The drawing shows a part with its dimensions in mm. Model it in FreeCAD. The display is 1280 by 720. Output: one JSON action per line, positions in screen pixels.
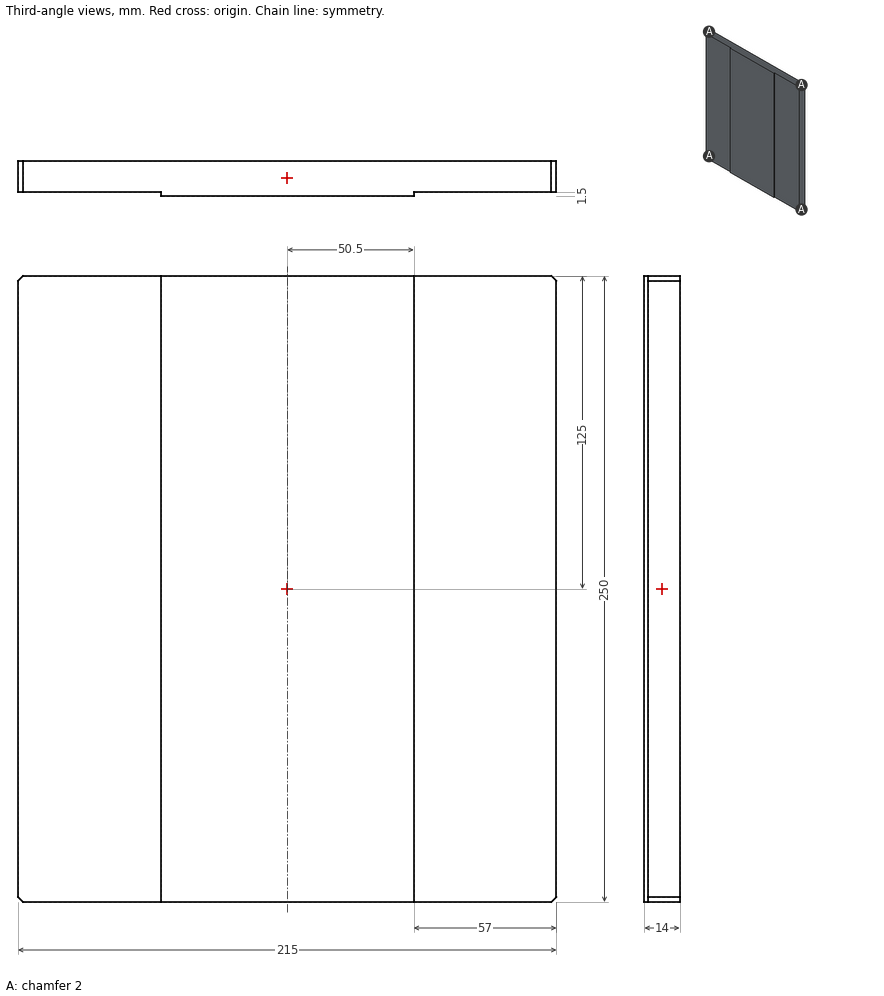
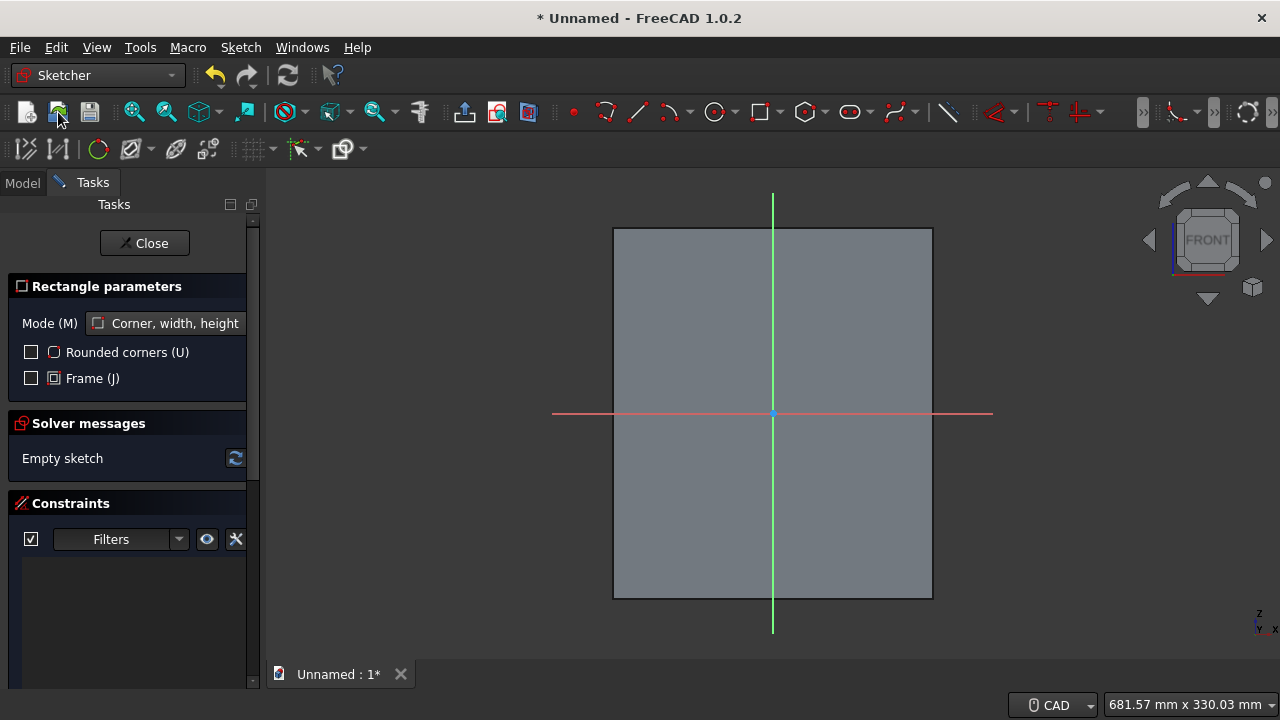
{"action": "left_click", "coordinate": [848, 228]}
{"action": "left_click", "coordinate": [933, 599]}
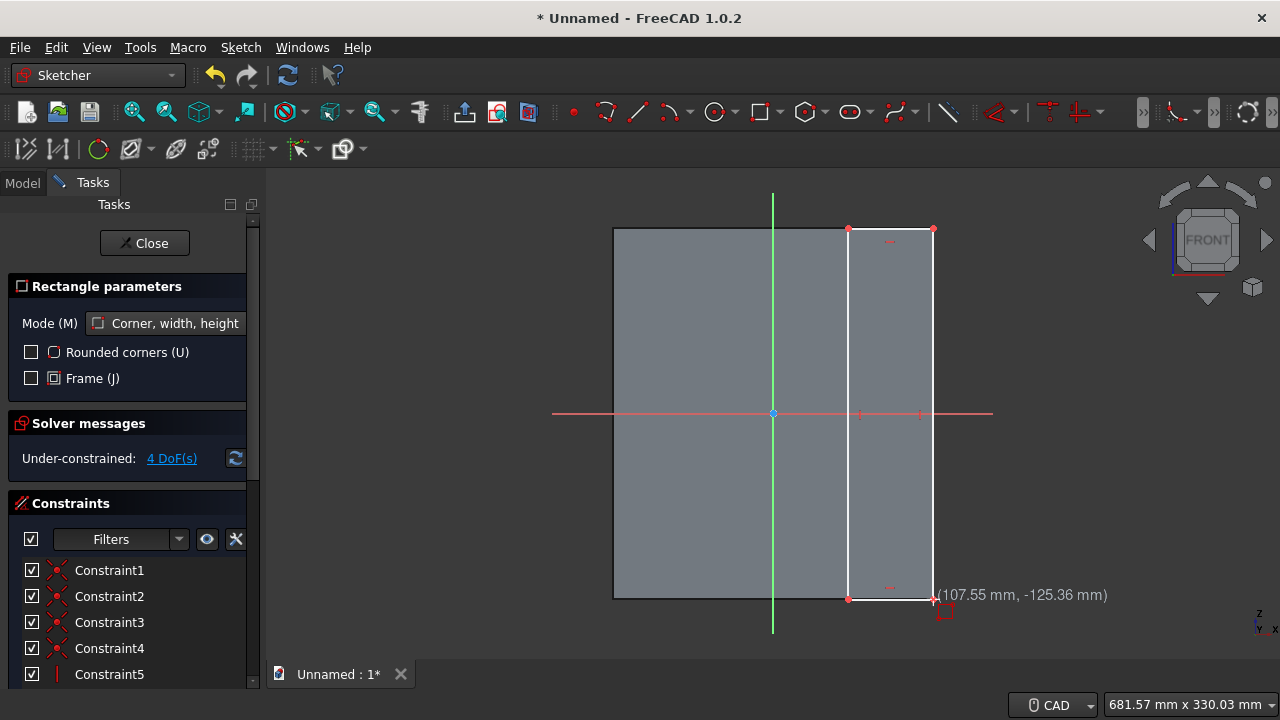
{"action": "left_click", "coordinate": [613, 228]}
{"action": "left_click", "coordinate": [698, 599]}
{"action": "key", "text": "Escape"}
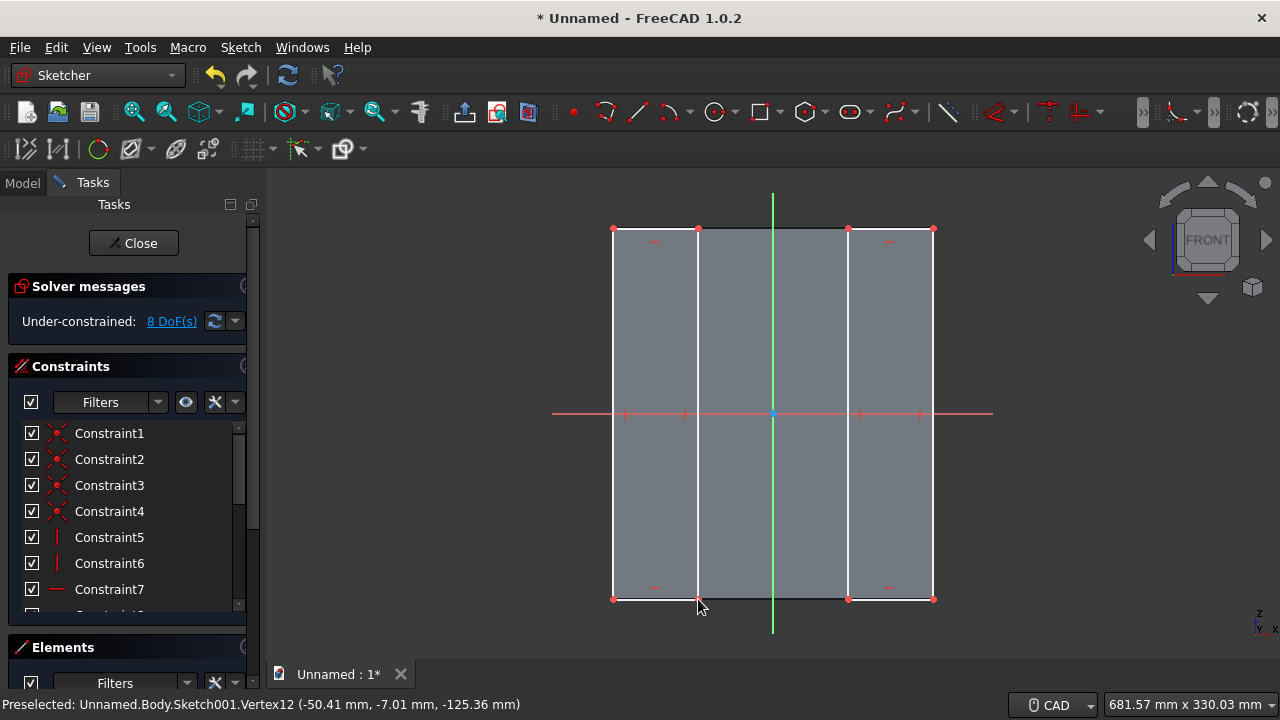
{"action": "left_click", "coordinate": [933, 229]}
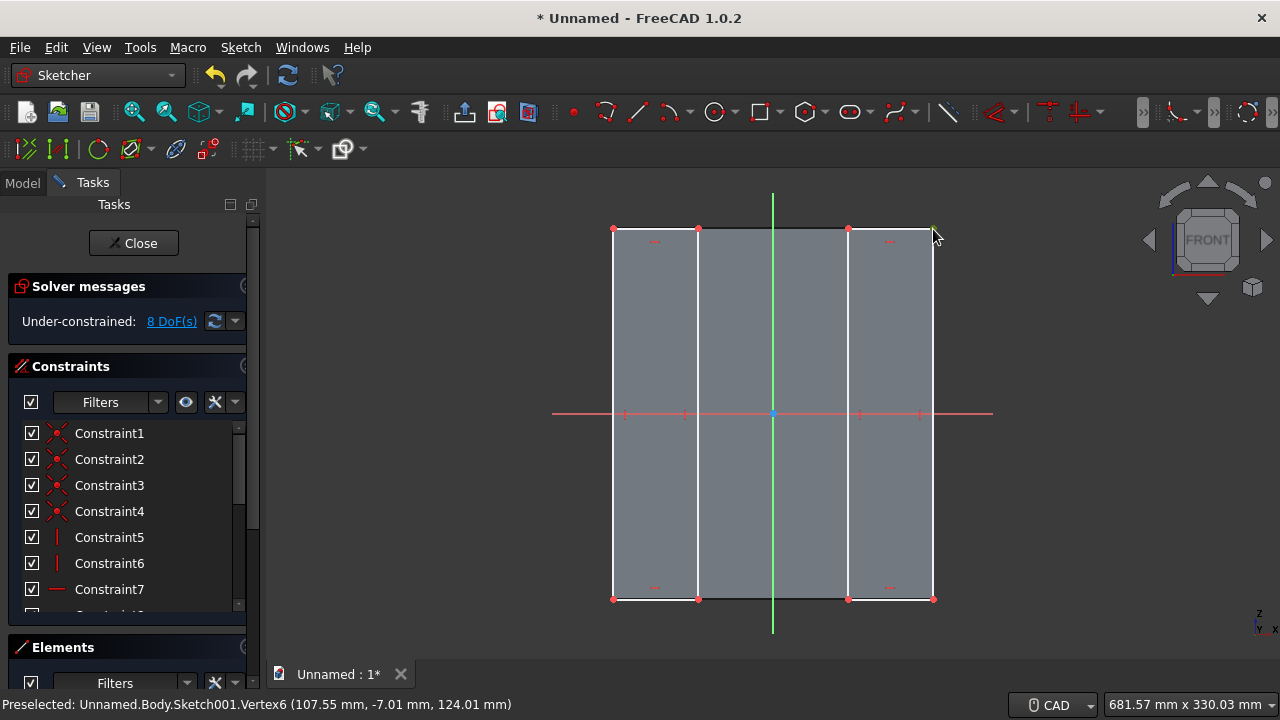
{"action": "left_click", "coordinate": [613, 229]}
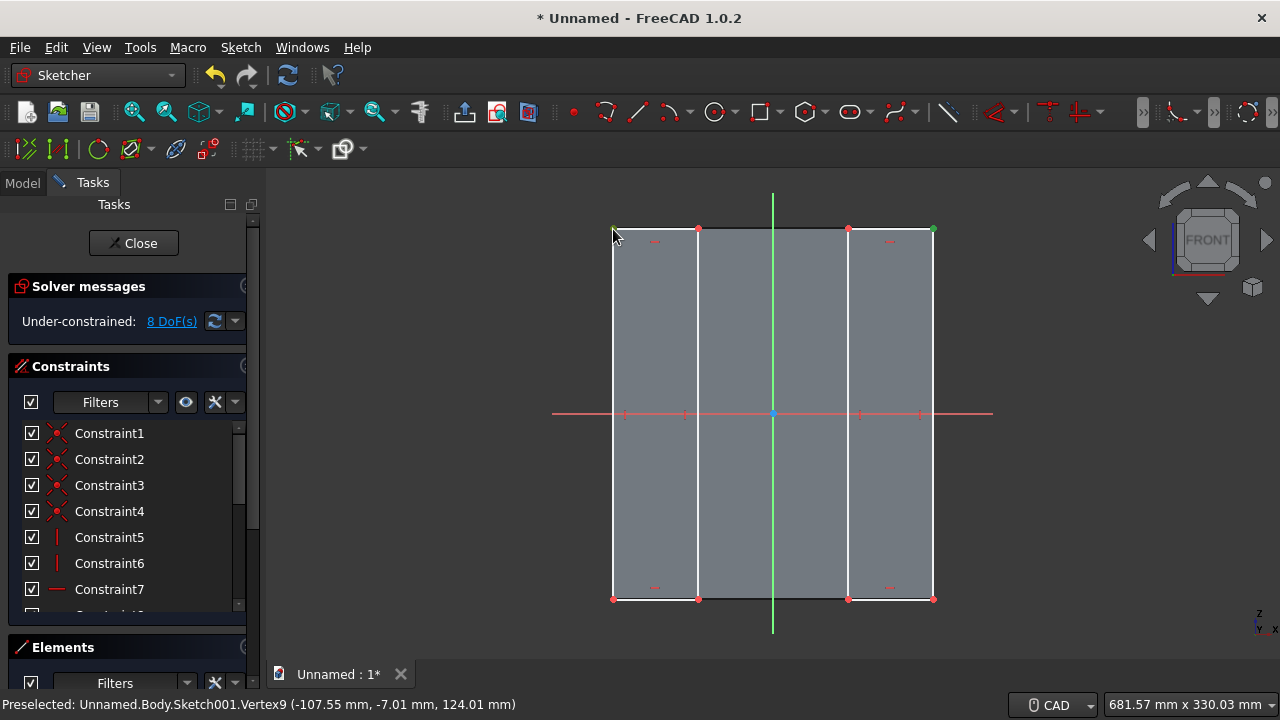
{"action": "left_click", "coordinate": [773, 600]}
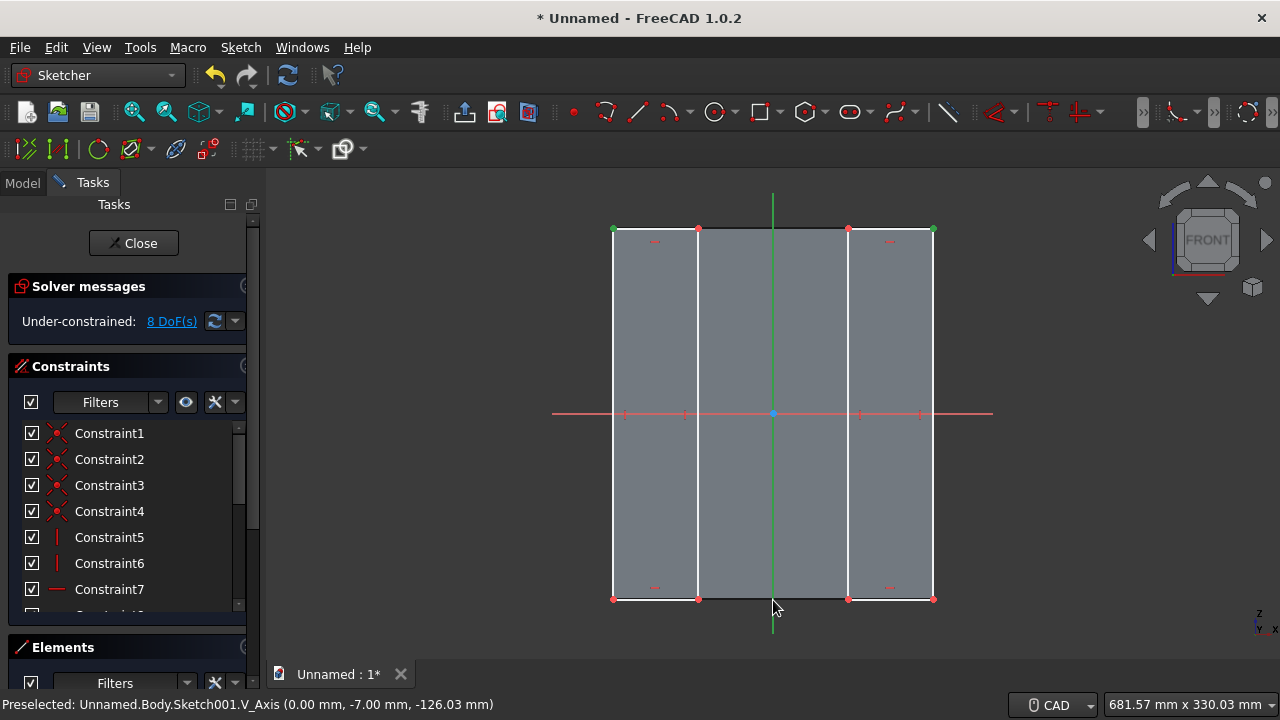
{"action": "key", "text": "s"}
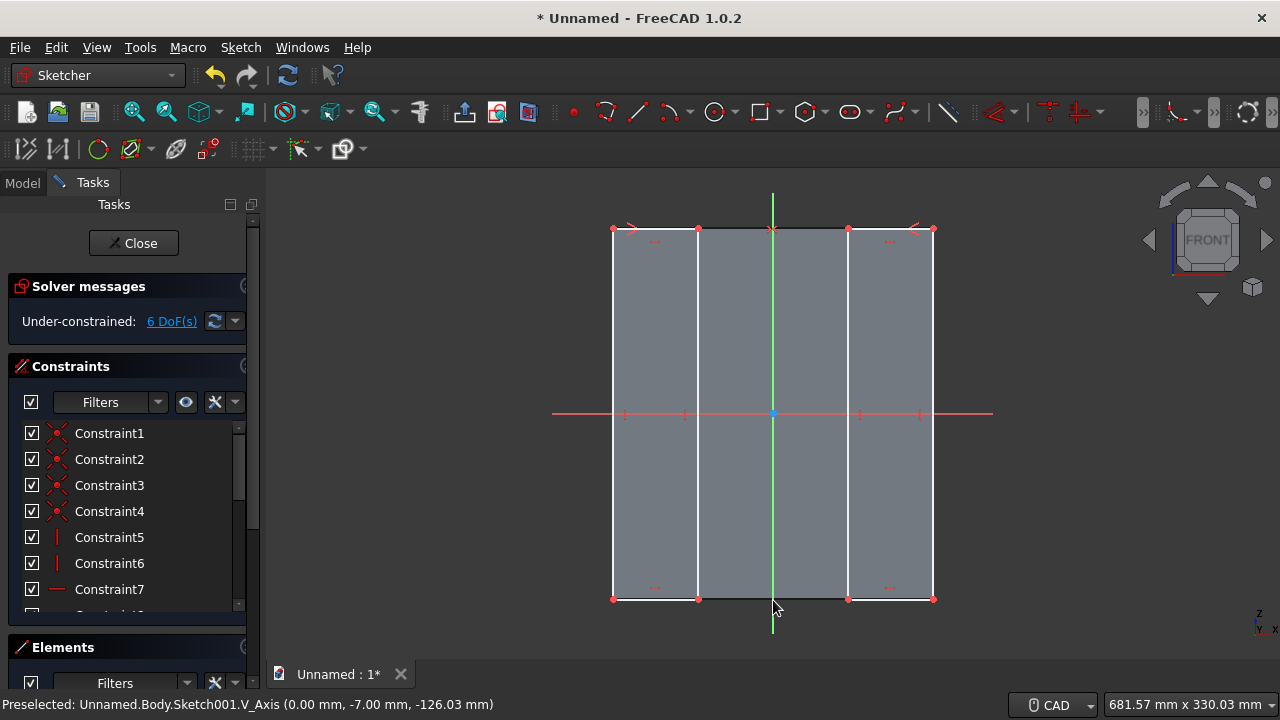
{"action": "left_click", "coordinate": [848, 600]}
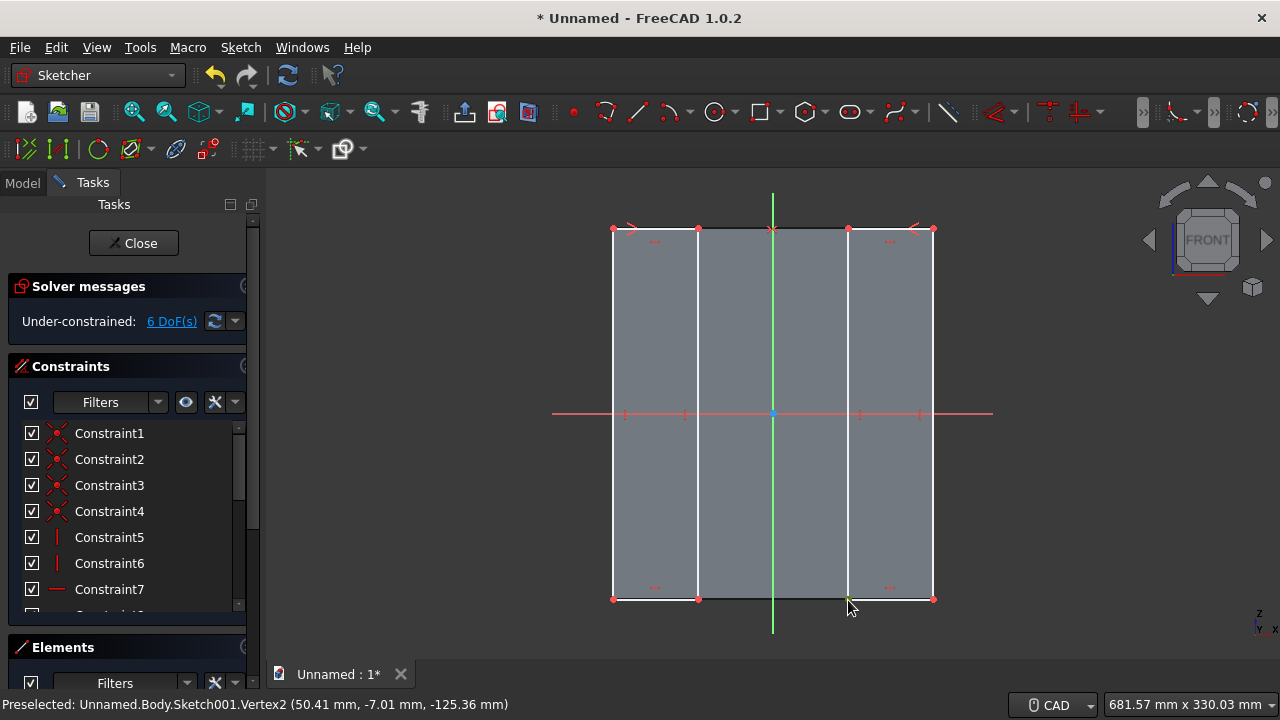
{"action": "left_click", "coordinate": [698, 600]}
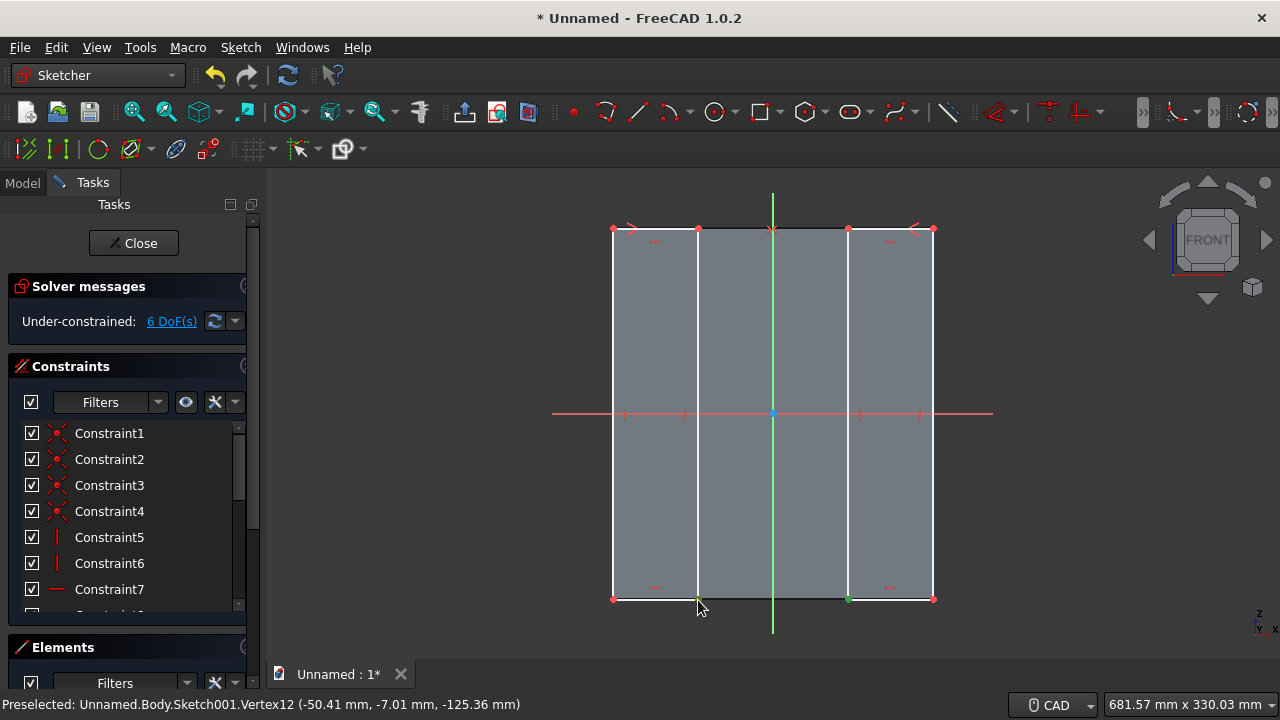
{"action": "left_click", "coordinate": [773, 600]}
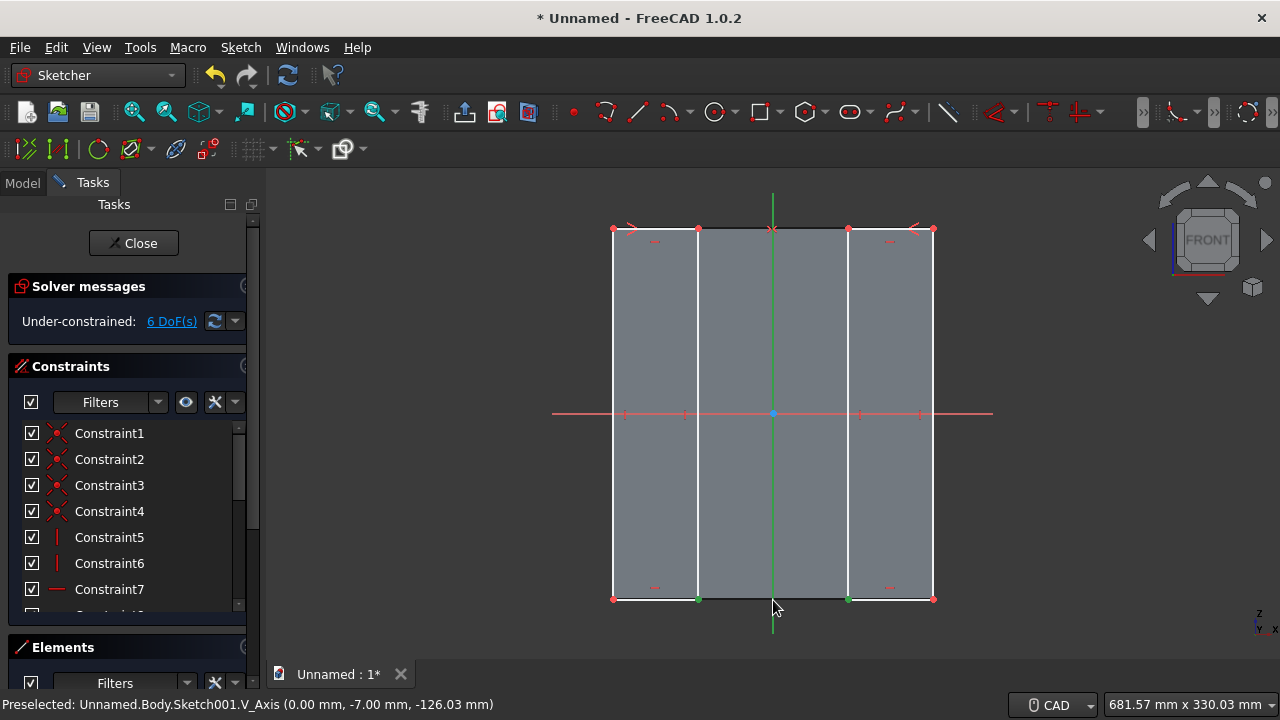
{"action": "key", "text": "s"}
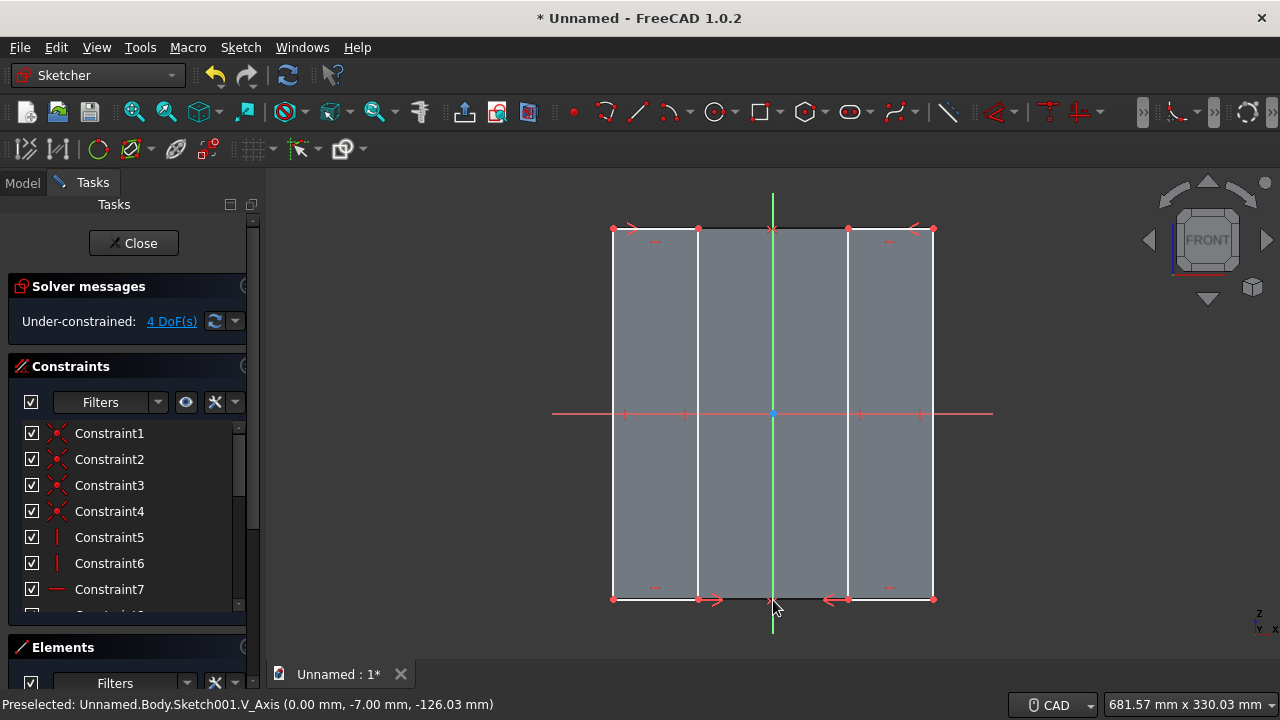
{"action": "left_click", "coordinate": [873, 600]}